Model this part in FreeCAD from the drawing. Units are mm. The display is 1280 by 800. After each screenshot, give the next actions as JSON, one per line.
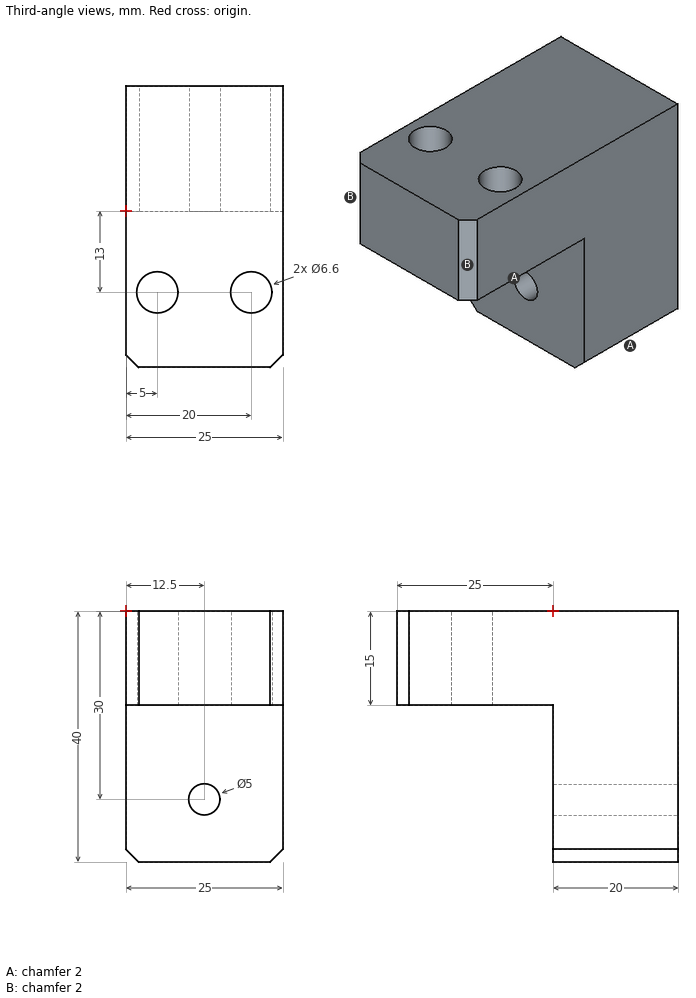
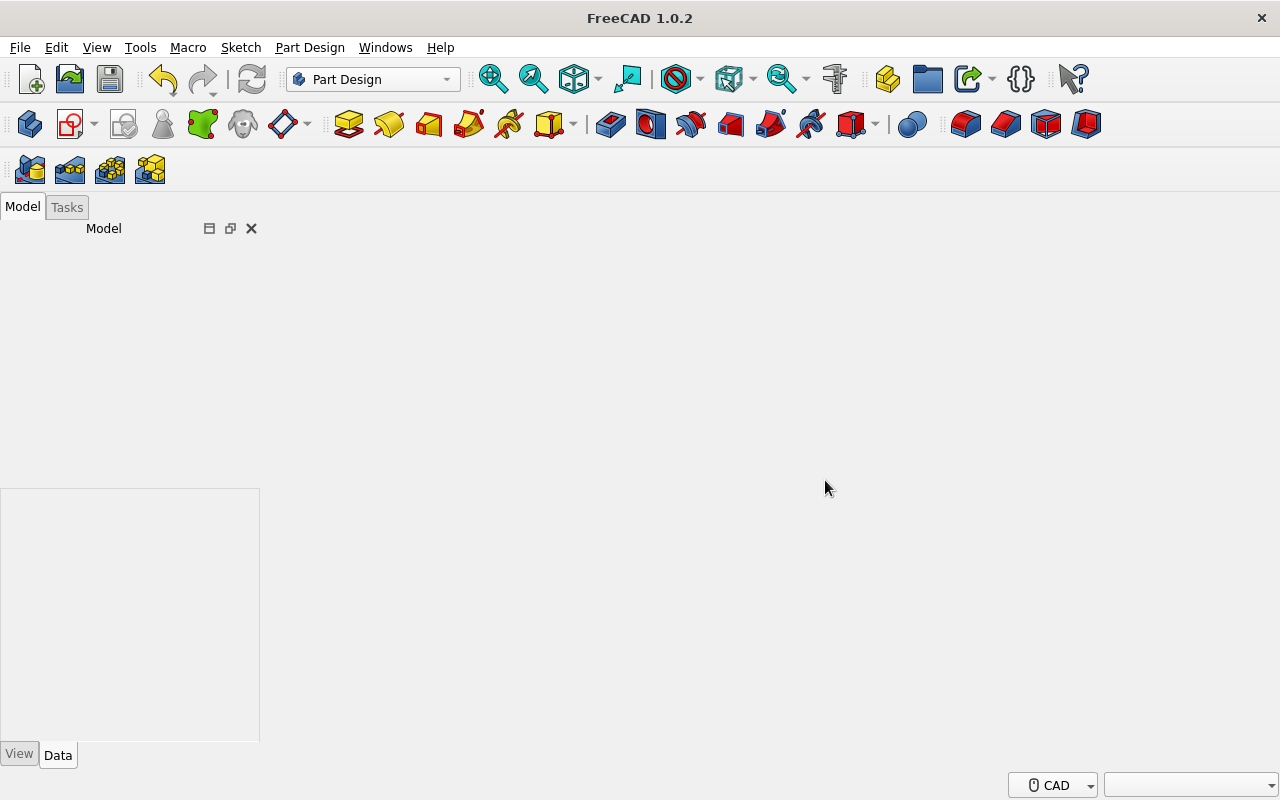
{"action": "left_click", "coordinate": [30, 80]}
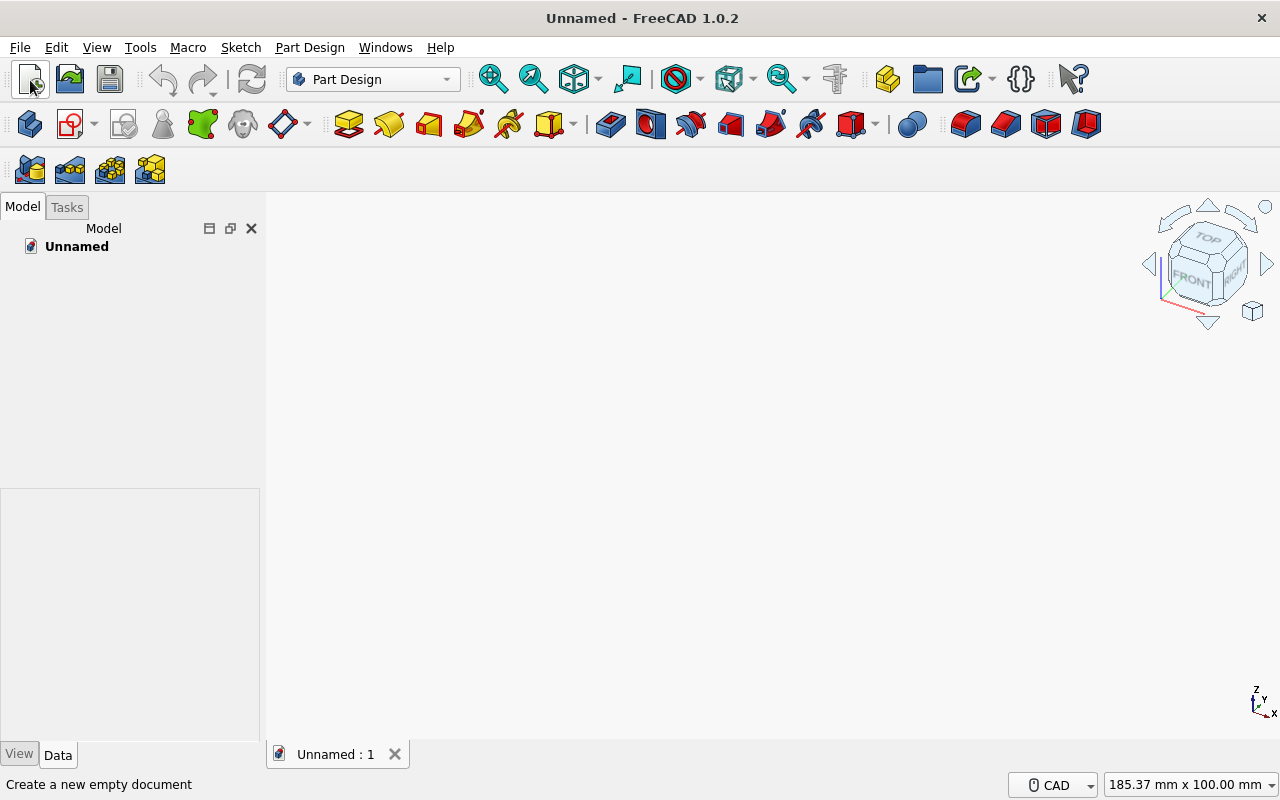
{"action": "left_click", "coordinate": [70, 124]}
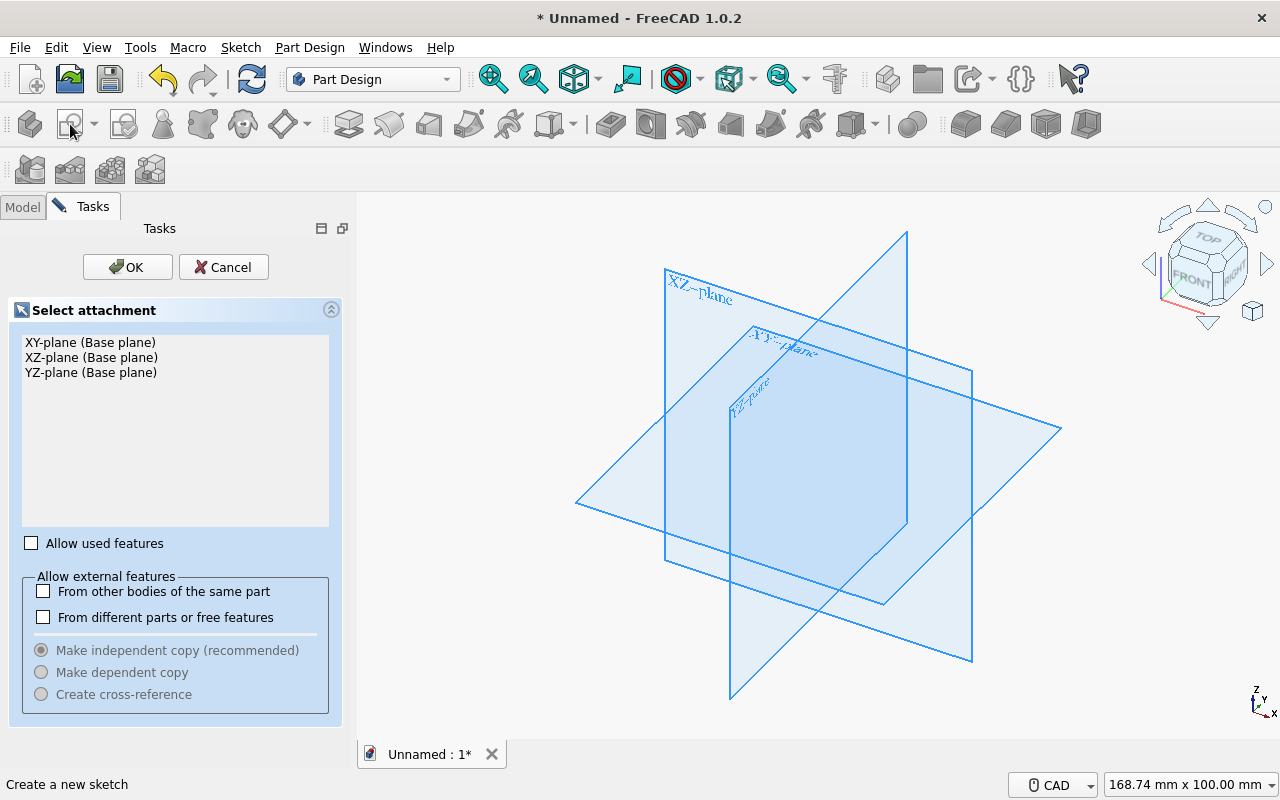
{"action": "left_click", "coordinate": [82, 358]}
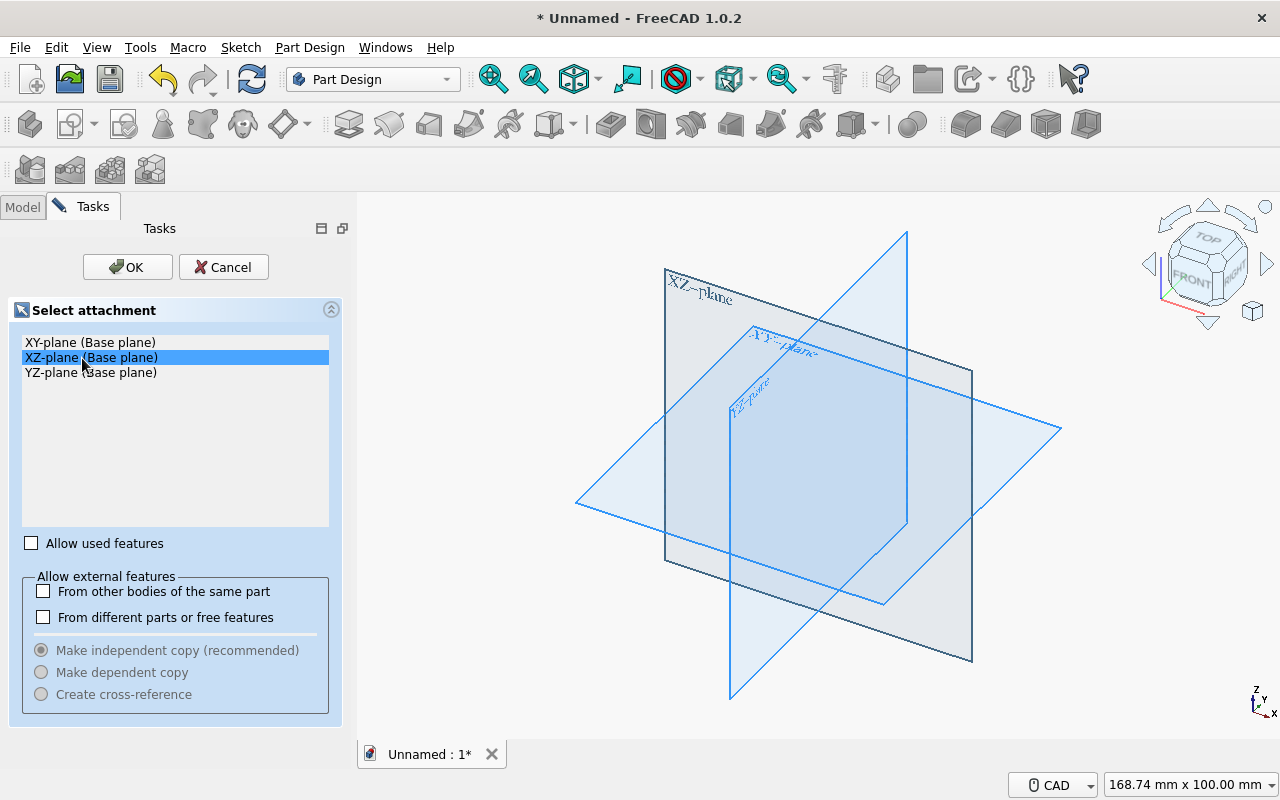
{"action": "left_click", "coordinate": [128, 267]}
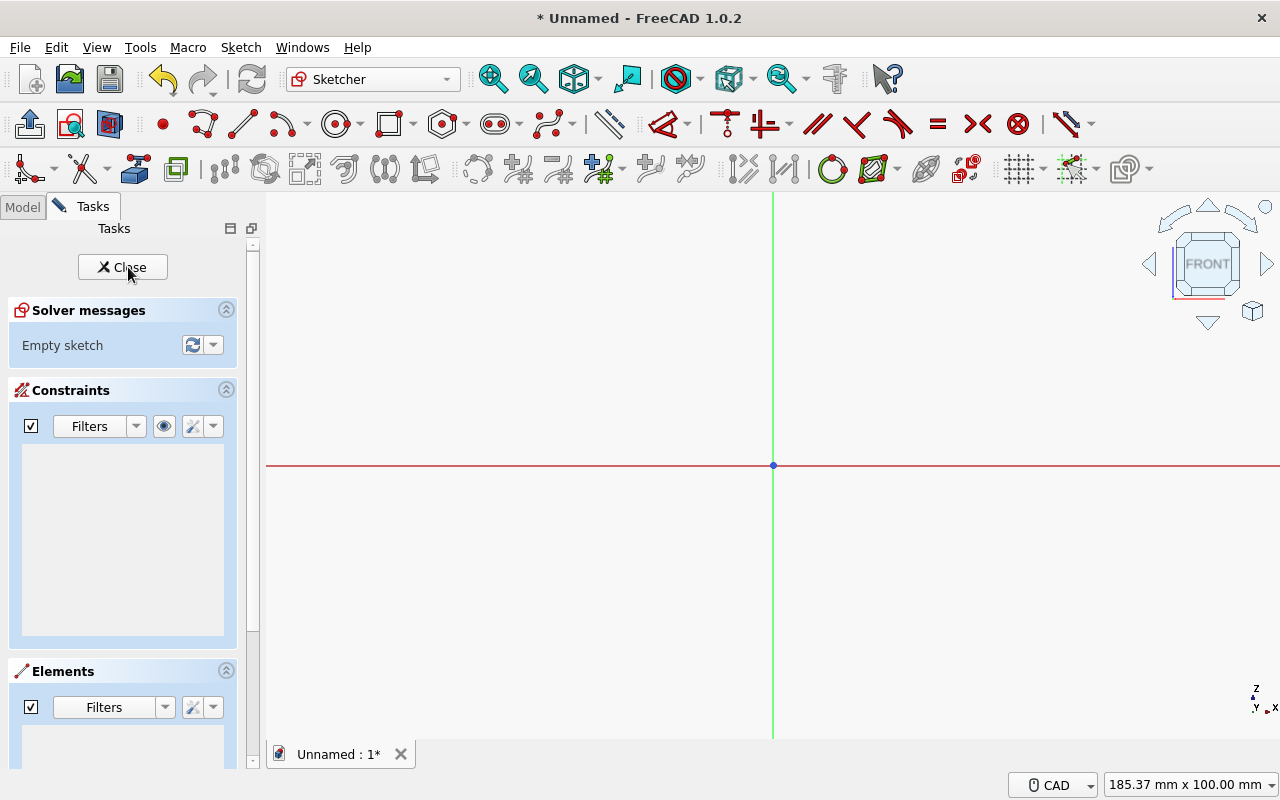
{"action": "scroll", "coordinate": [1115, 711], "scroll_direction": "up", "scroll_amount": 2}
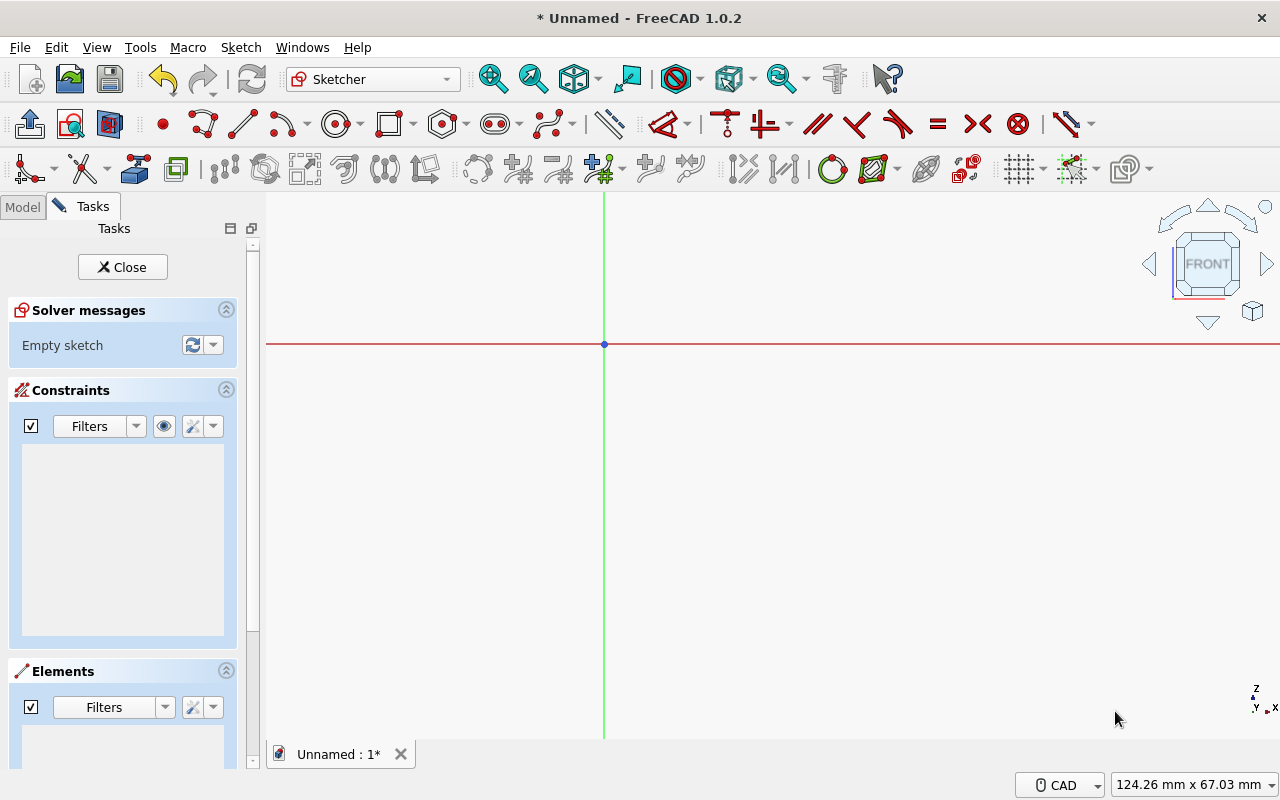
{"action": "key", "text": "g r"}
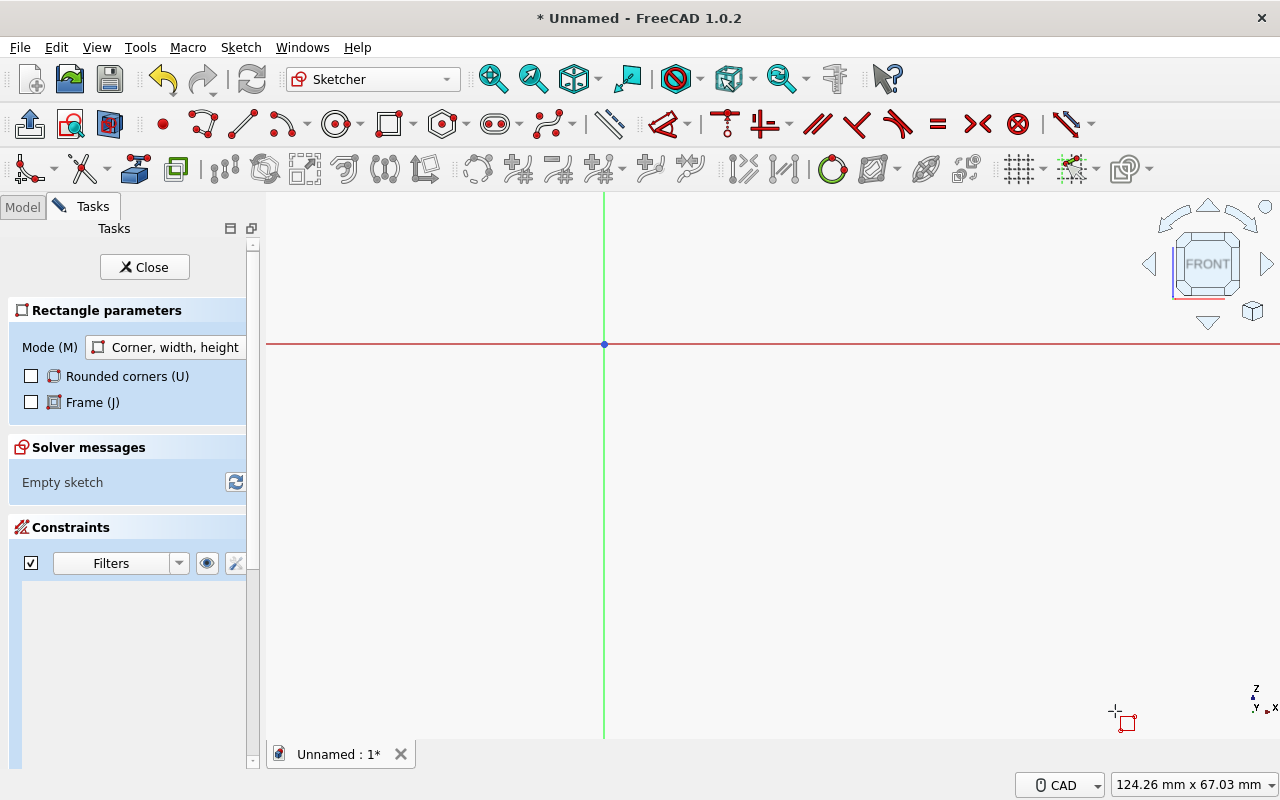
{"action": "left_click", "coordinate": [604, 344]}
{"action": "left_click", "coordinate": [808, 671]}
{"action": "key", "text": "Escape"}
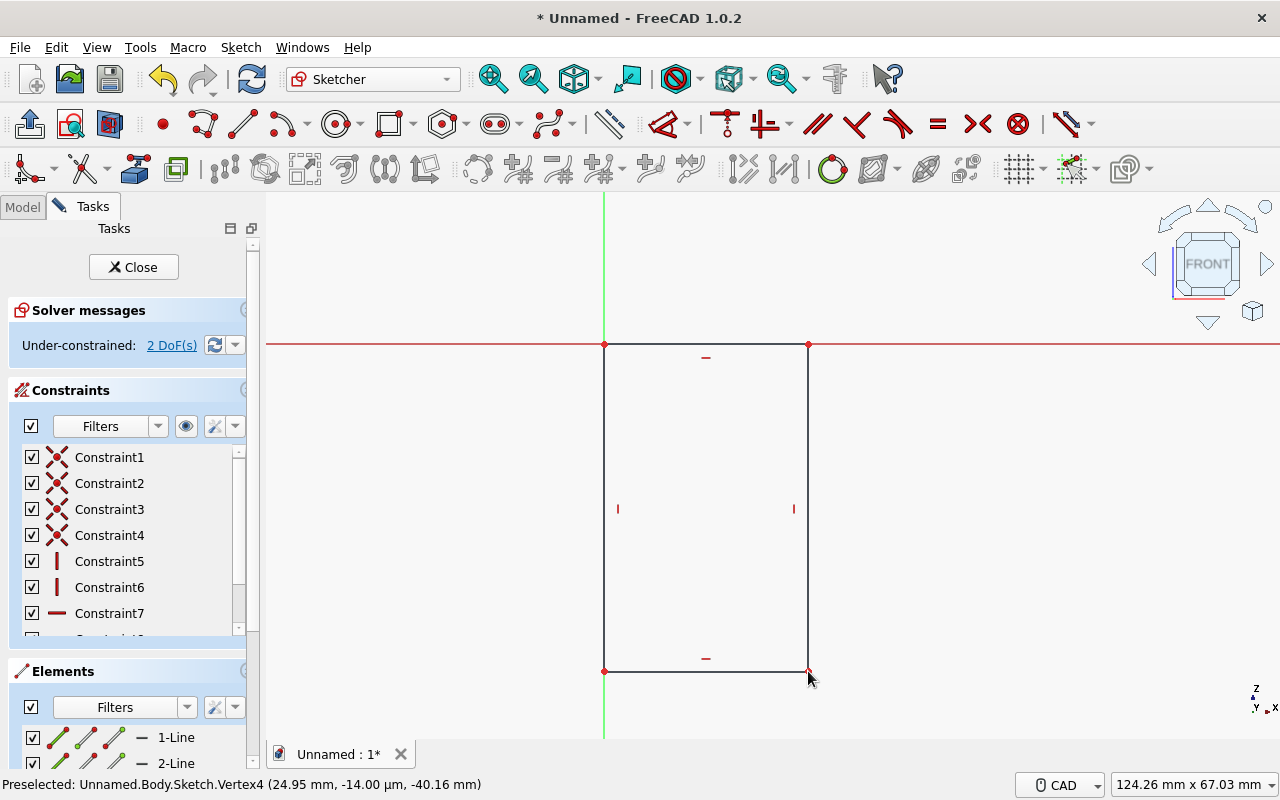
{"action": "left_click", "coordinate": [604, 443]}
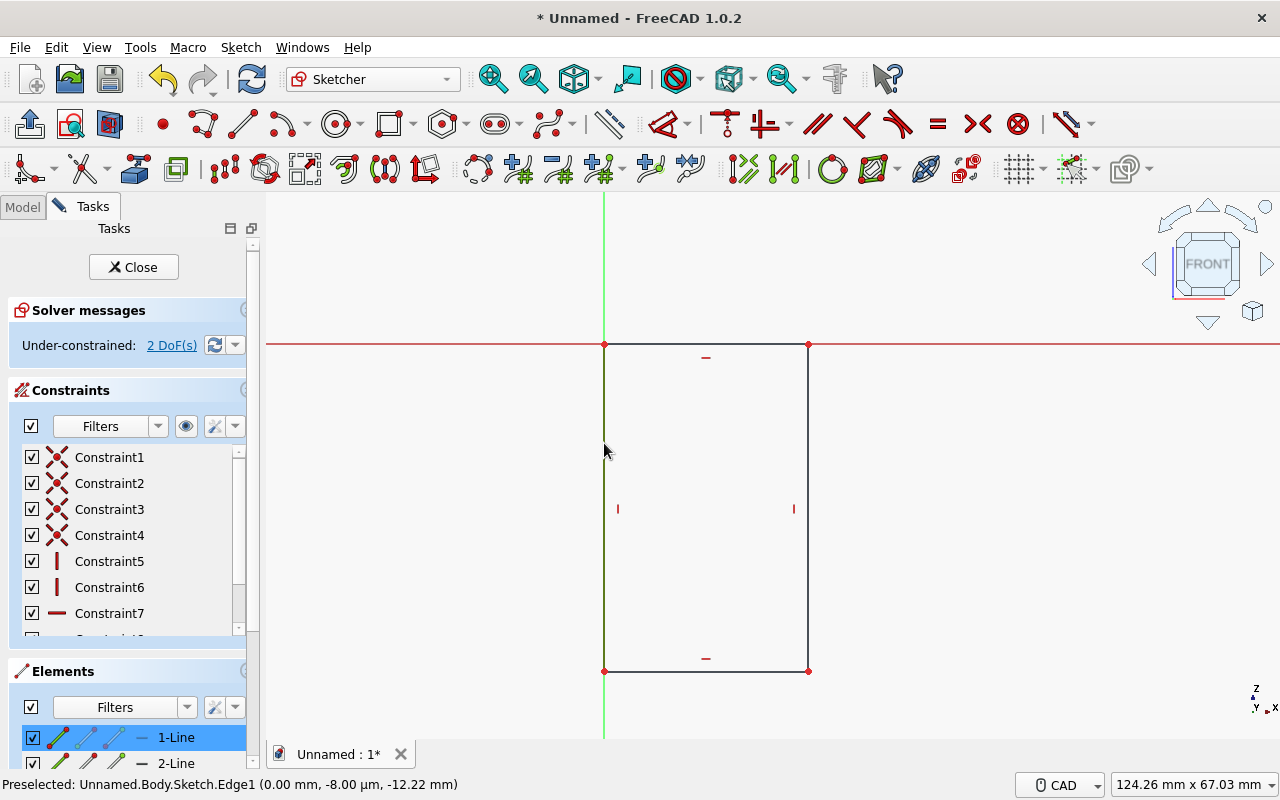
{"action": "key", "text": "i"}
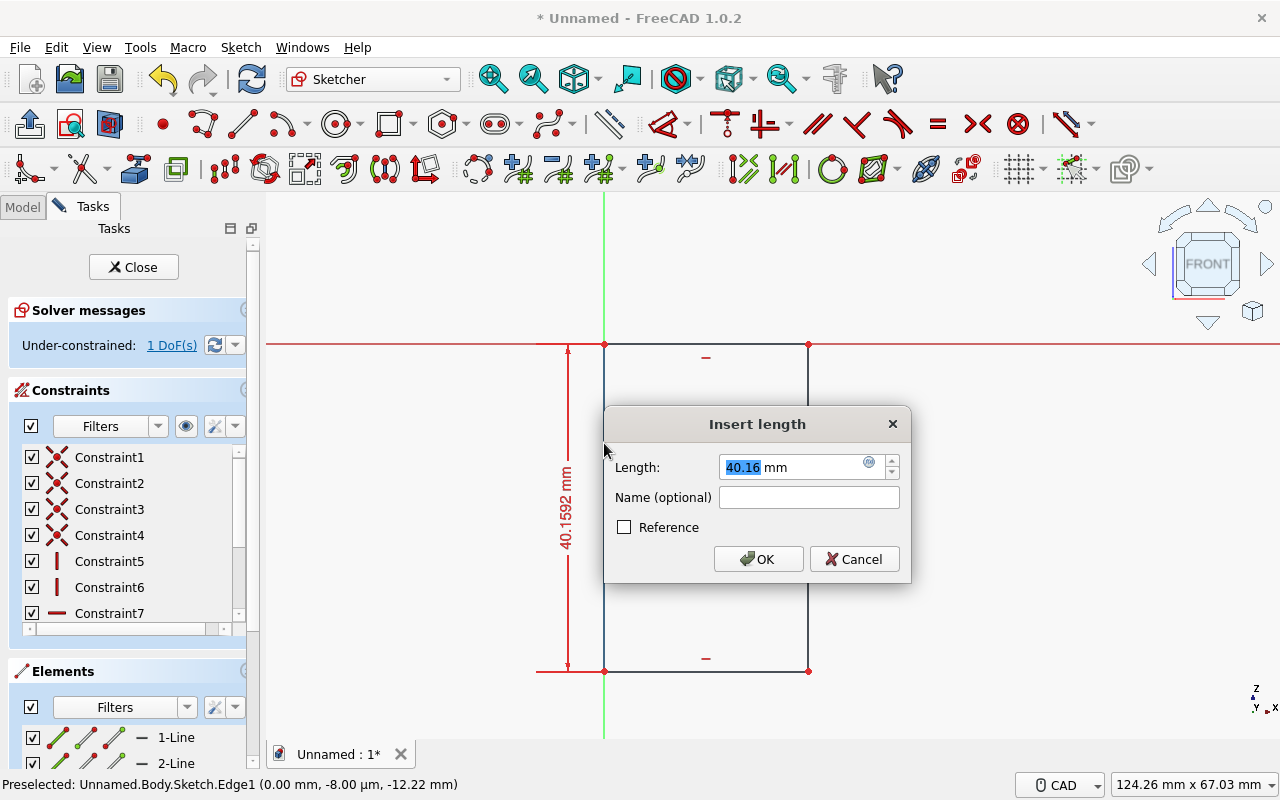
{"action": "type", "text": "40"}
{"action": "key", "text": "Return"}